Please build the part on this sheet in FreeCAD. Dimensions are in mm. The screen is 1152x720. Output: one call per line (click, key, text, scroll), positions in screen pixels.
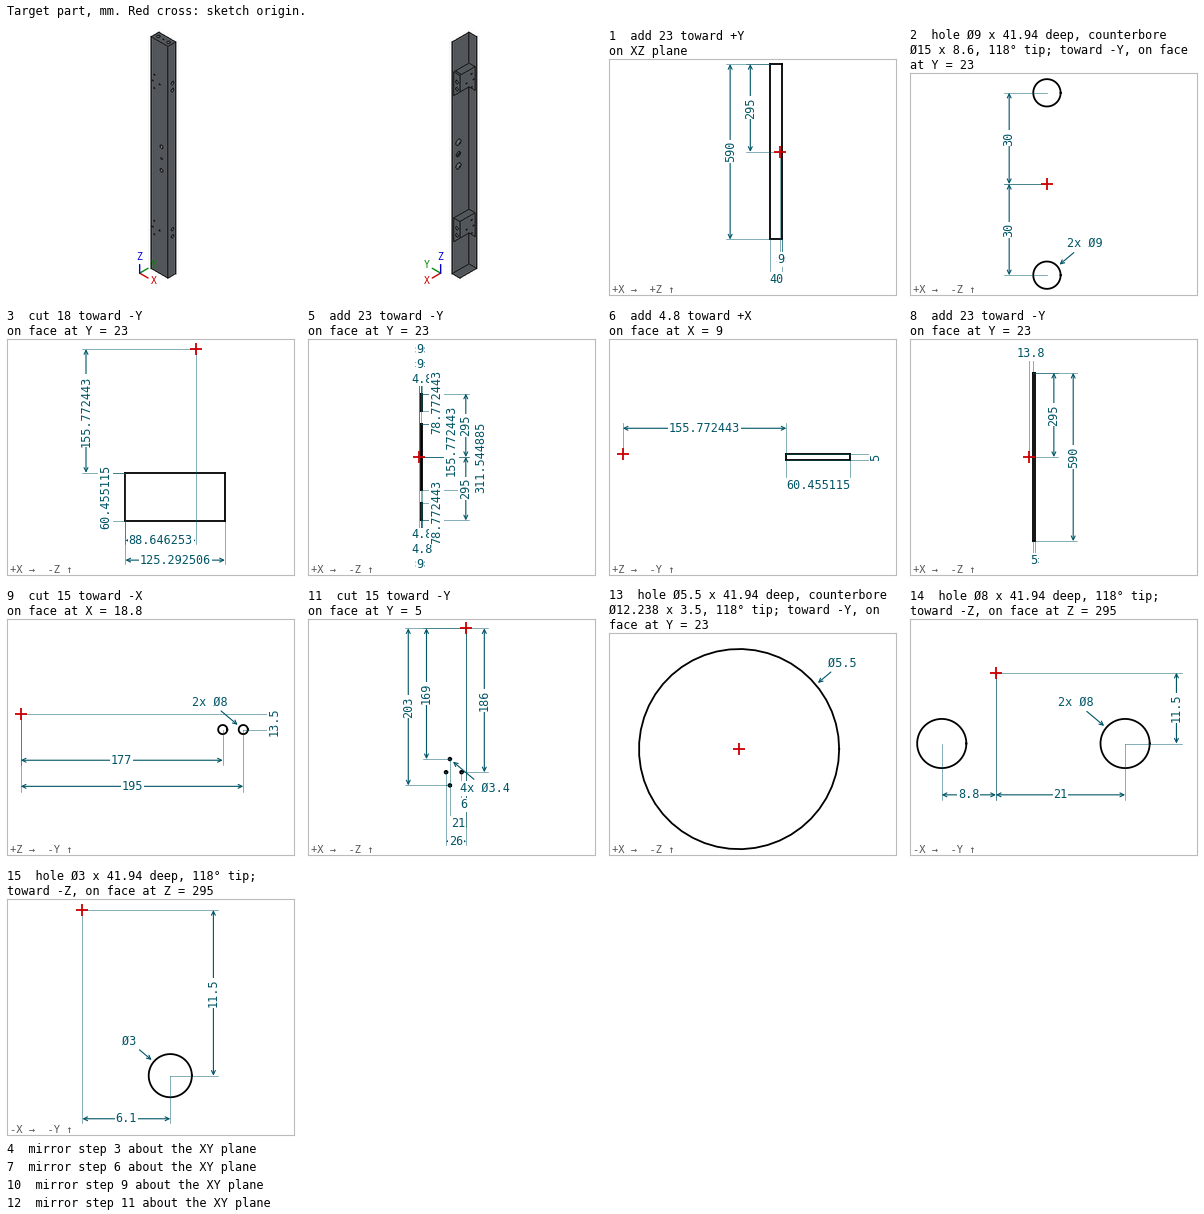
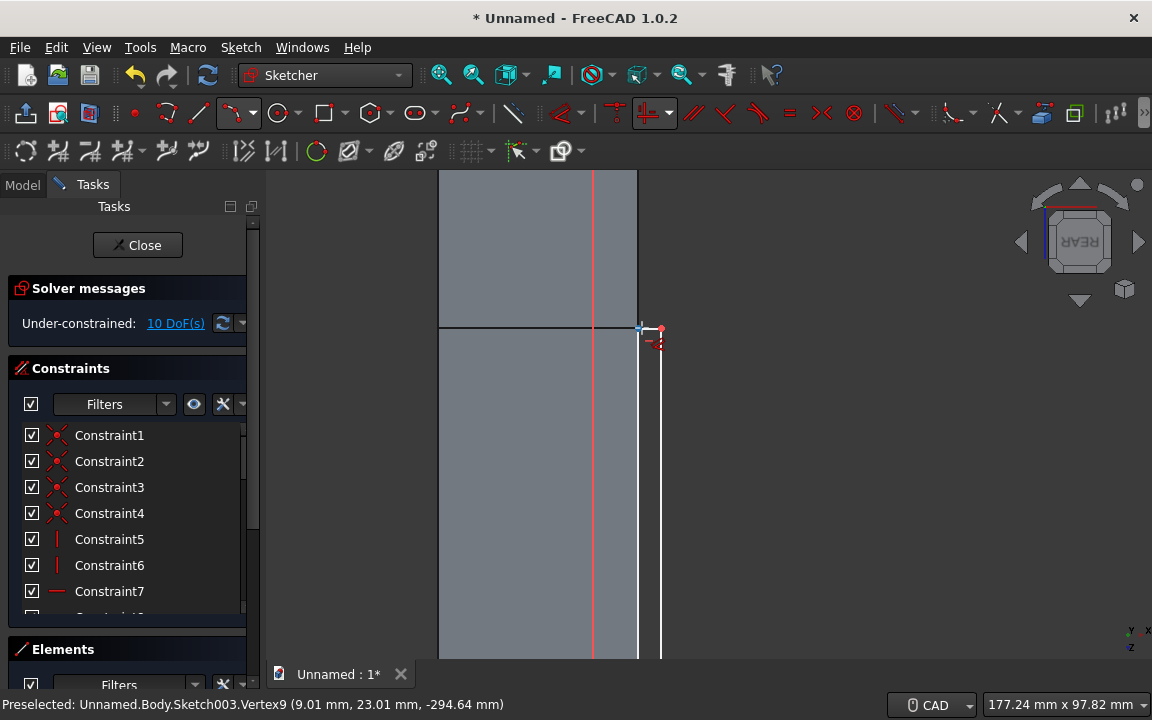
click(638, 329)
click(616, 295)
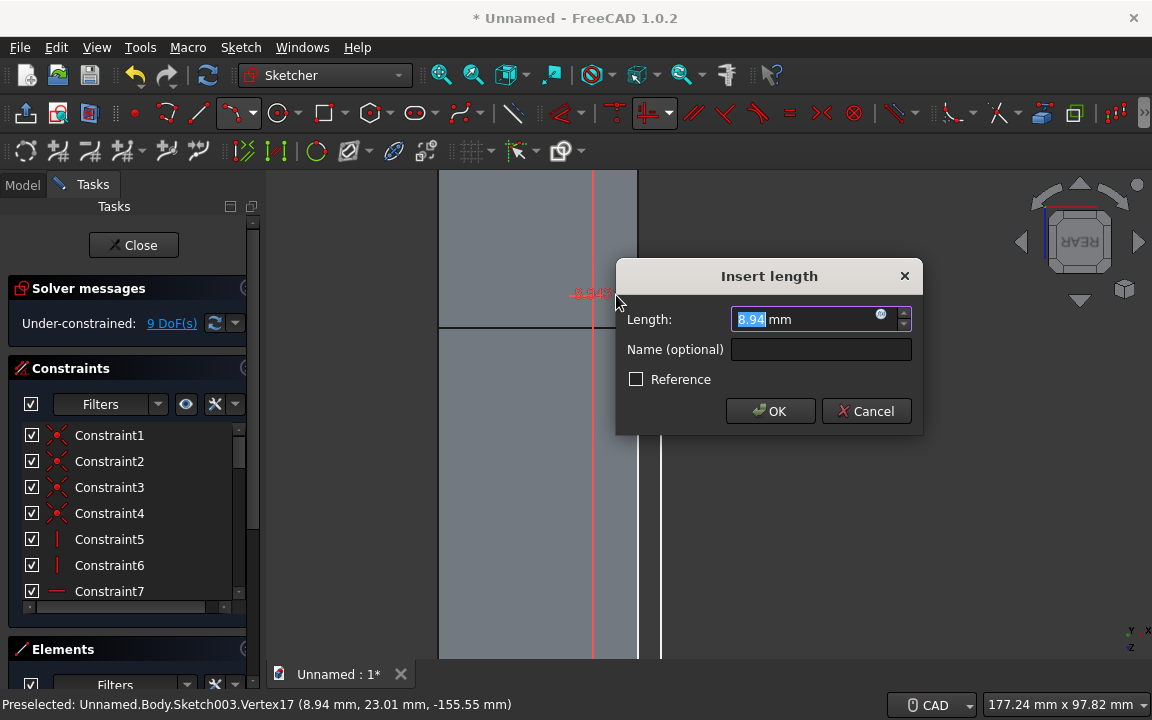
text(9)
key(Return)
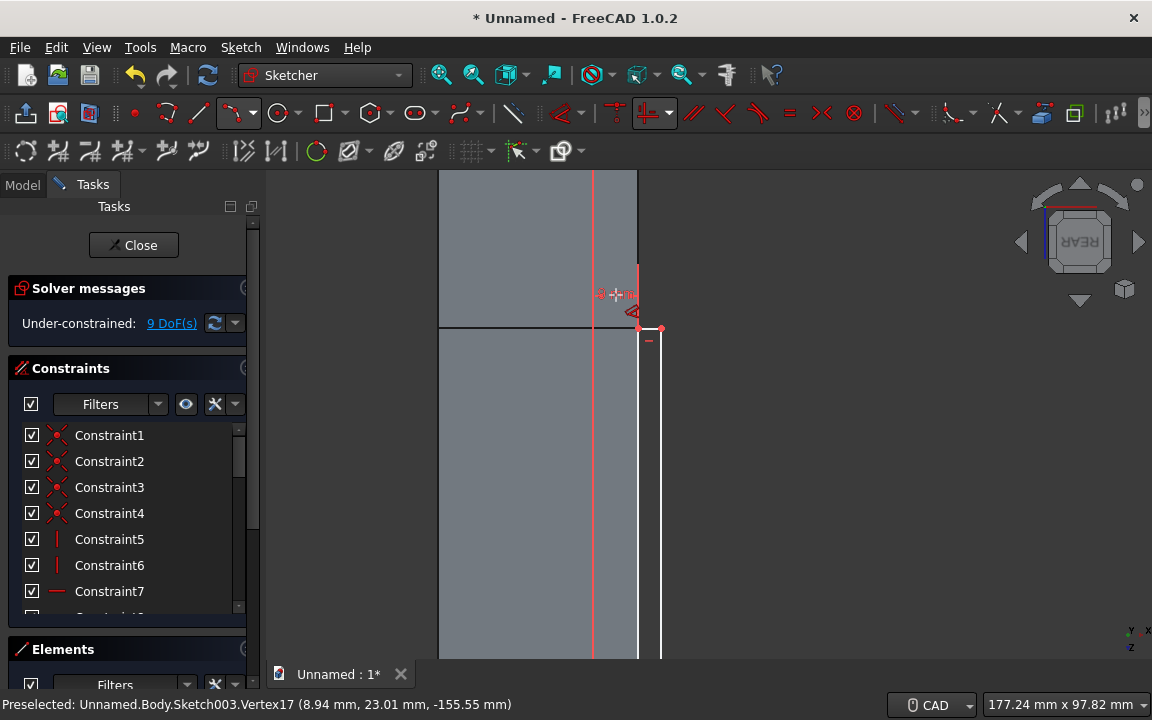
scroll(642, 328, down, 11)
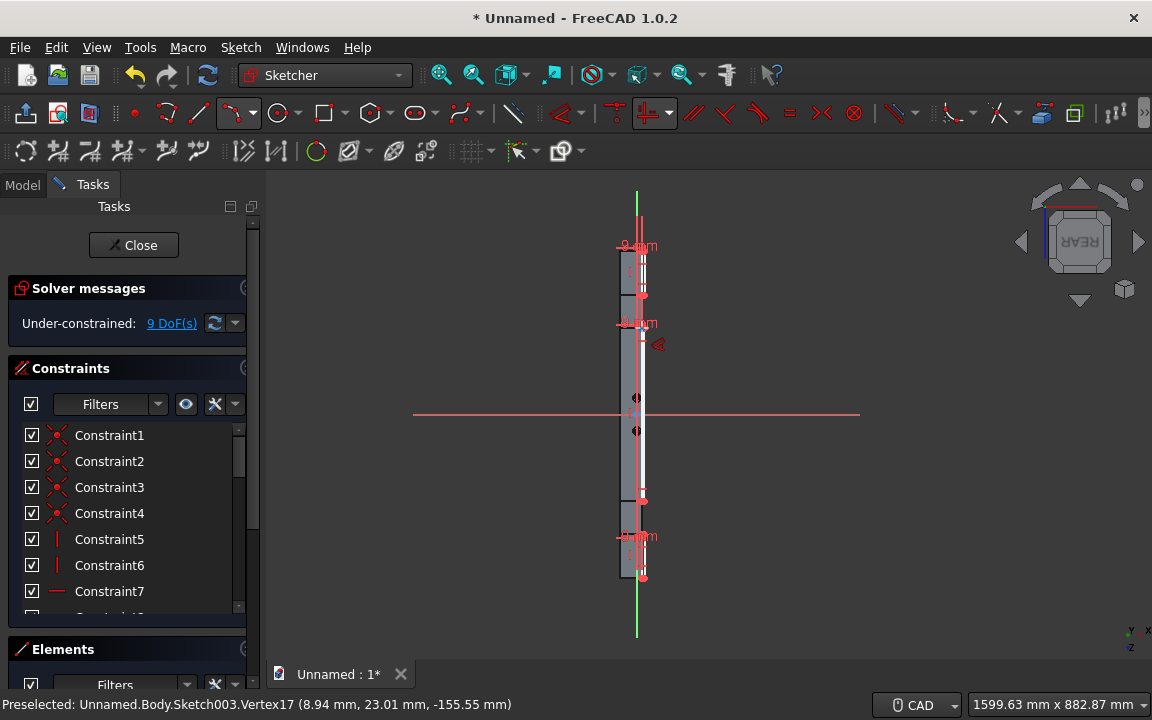
scroll(643, 578, up, 14)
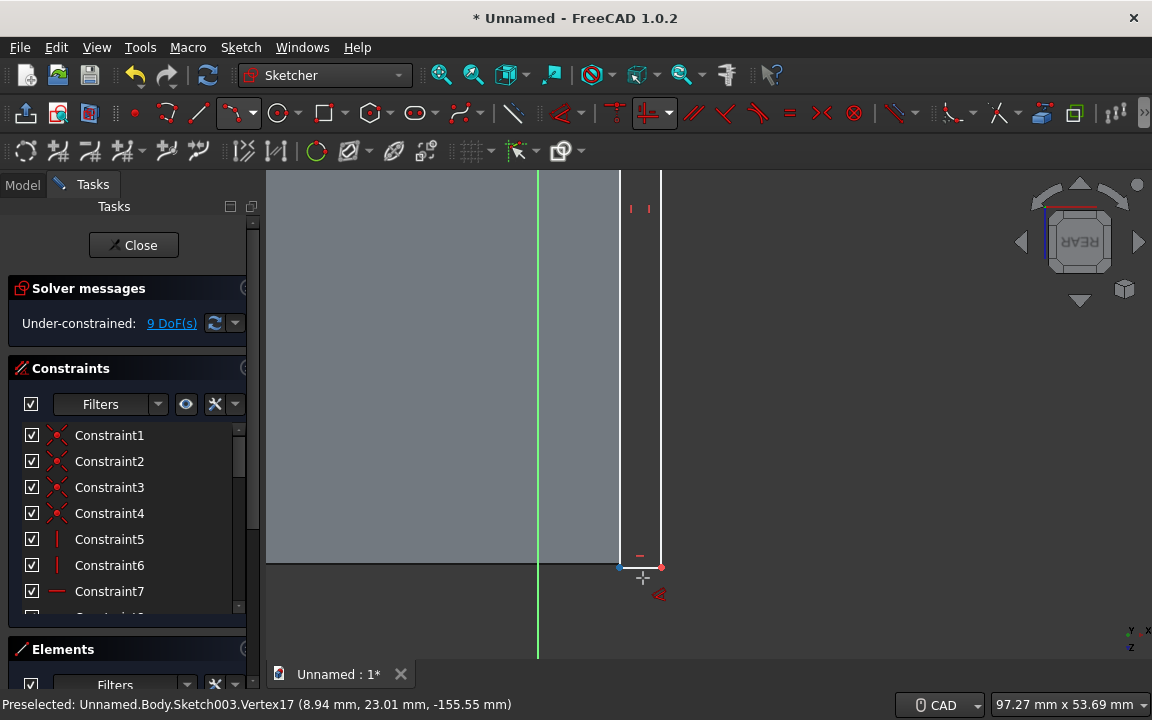
click(636, 568)
click(641, 602)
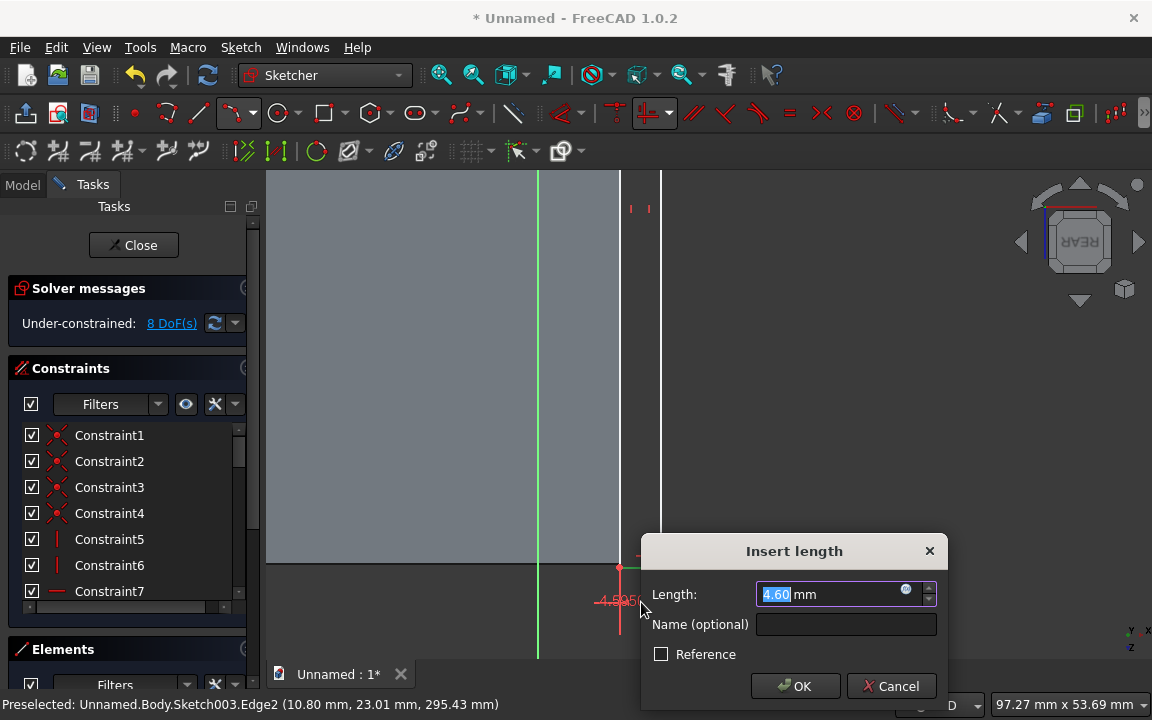
text(4.8)
key(Return)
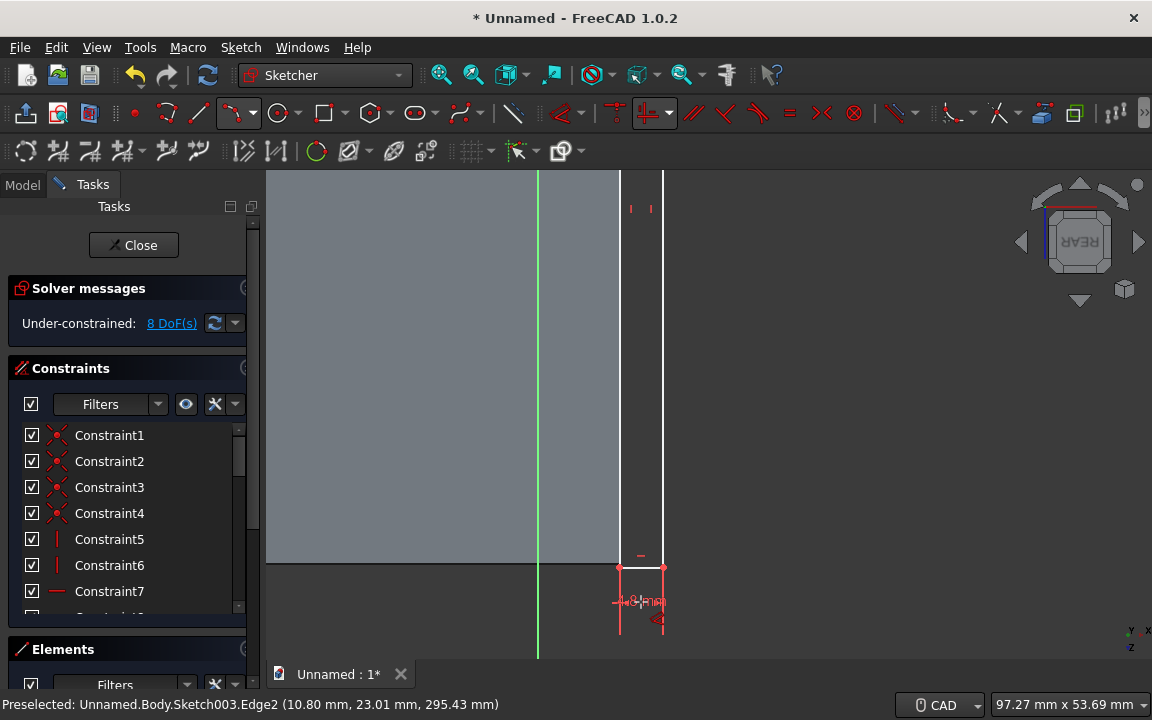
scroll(643, 579, down, 14)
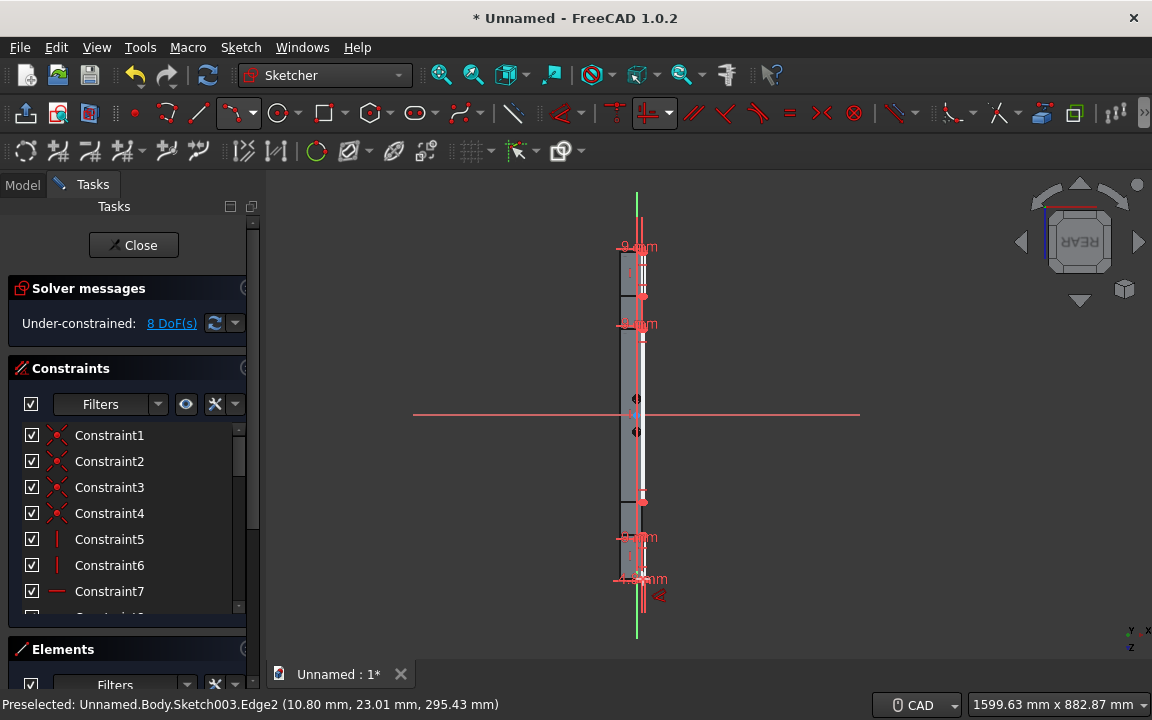
scroll(643, 296, up, 14)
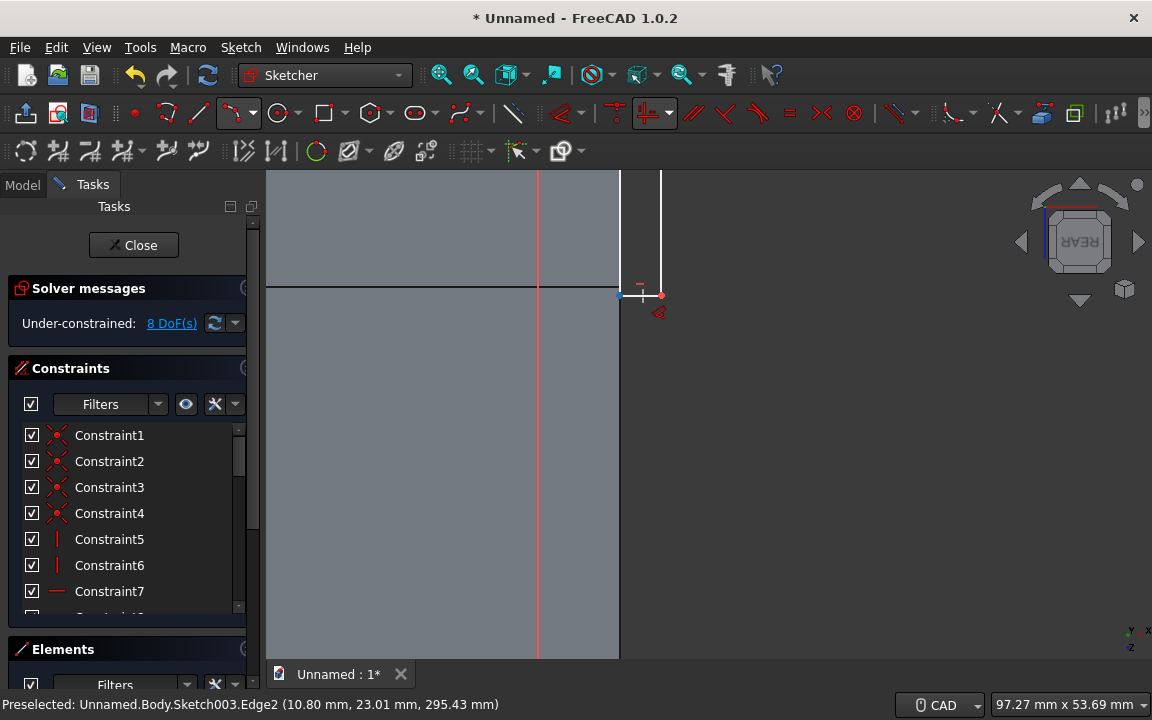
click(632, 296)
click(641, 262)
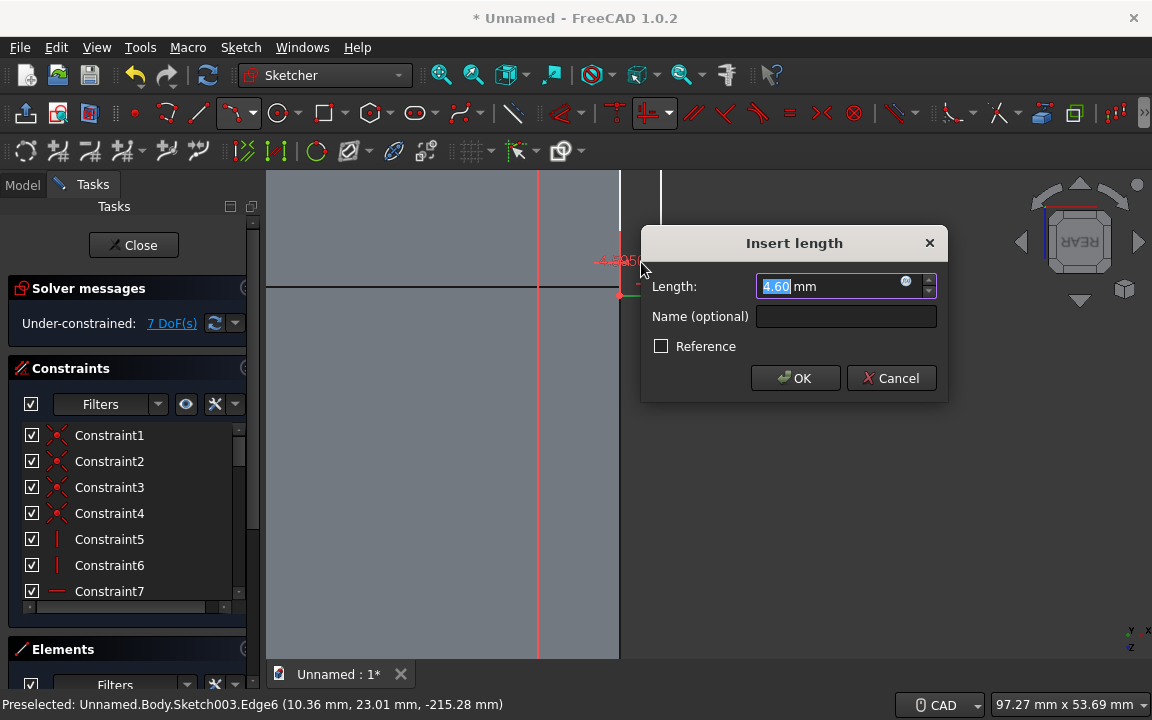
text(4.8)
key(Return)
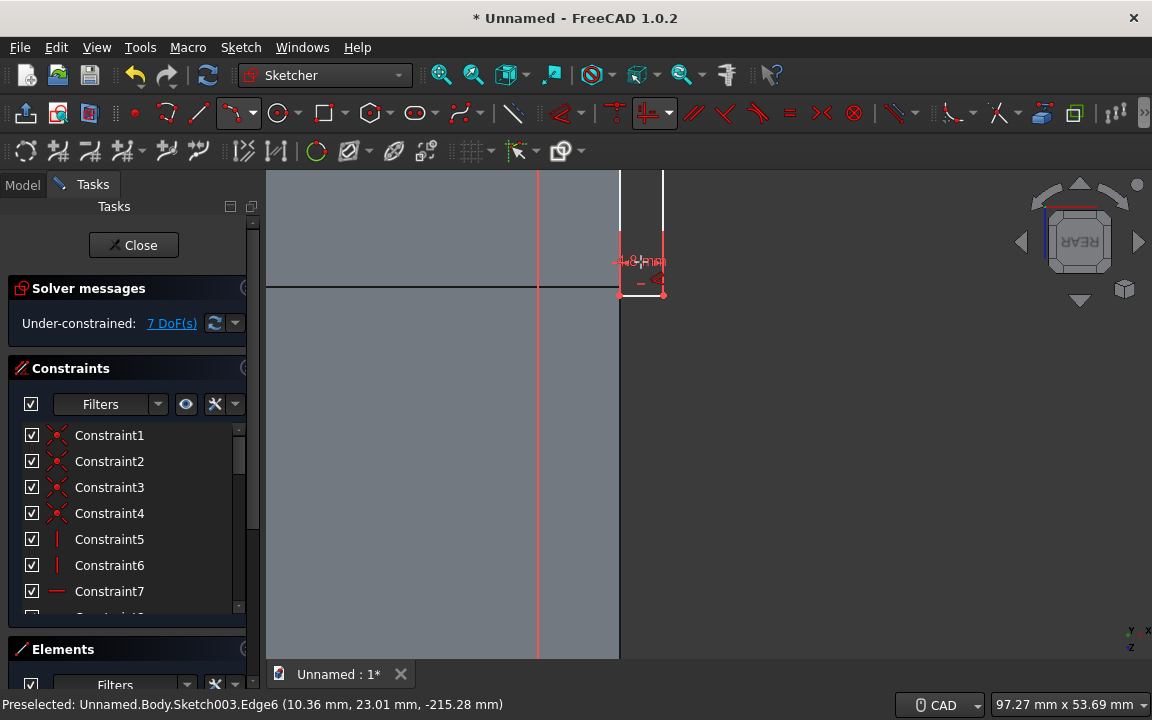
scroll(643, 295, down, 14)